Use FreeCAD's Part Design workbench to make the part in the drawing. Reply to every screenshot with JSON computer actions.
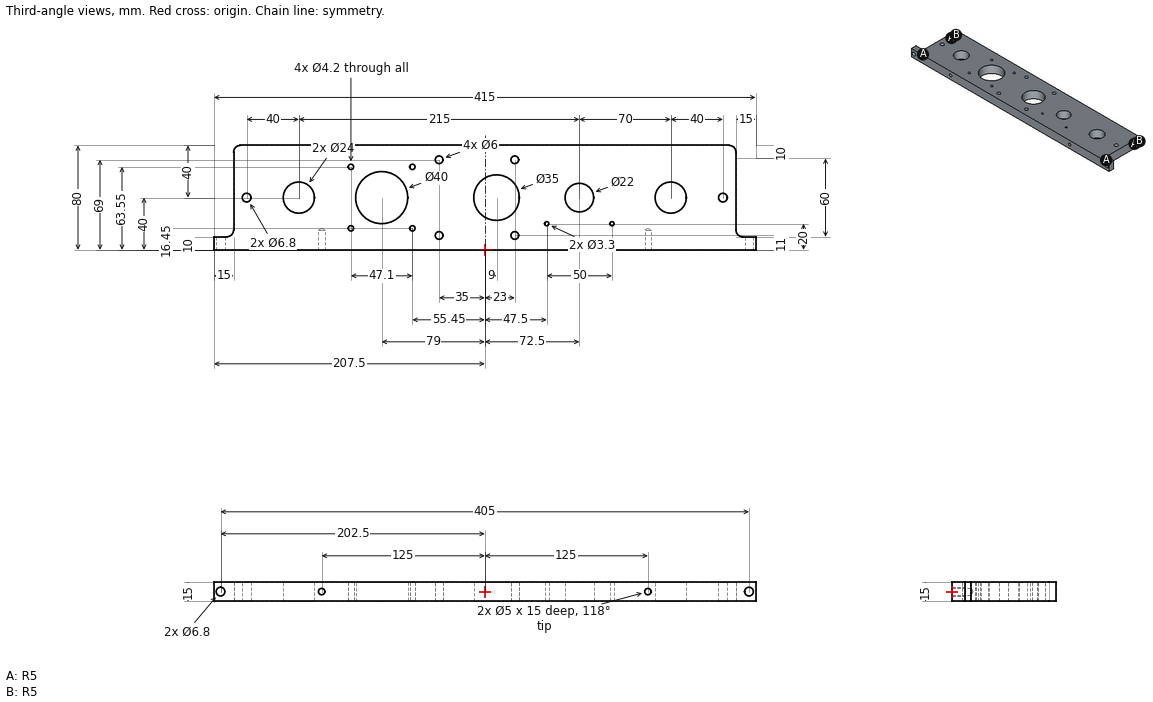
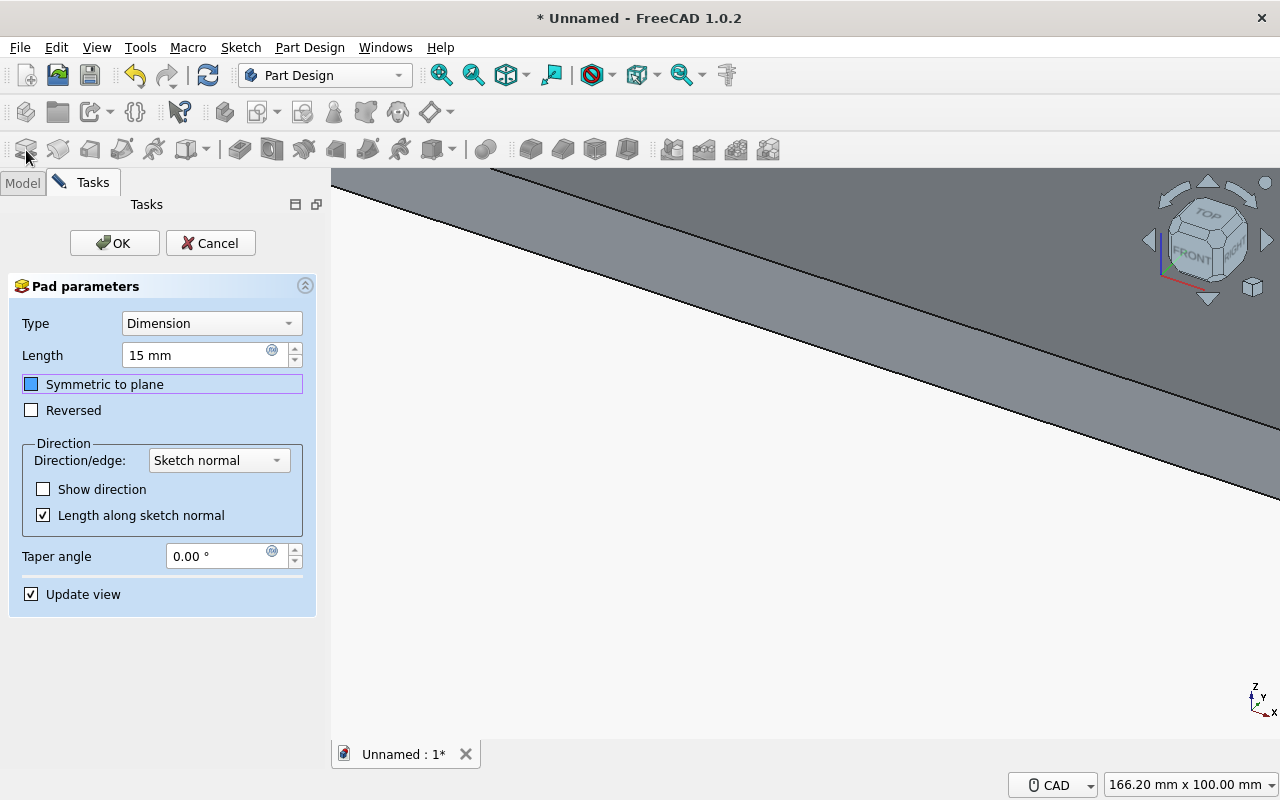
{"action": "left_click", "coordinate": [30, 384]}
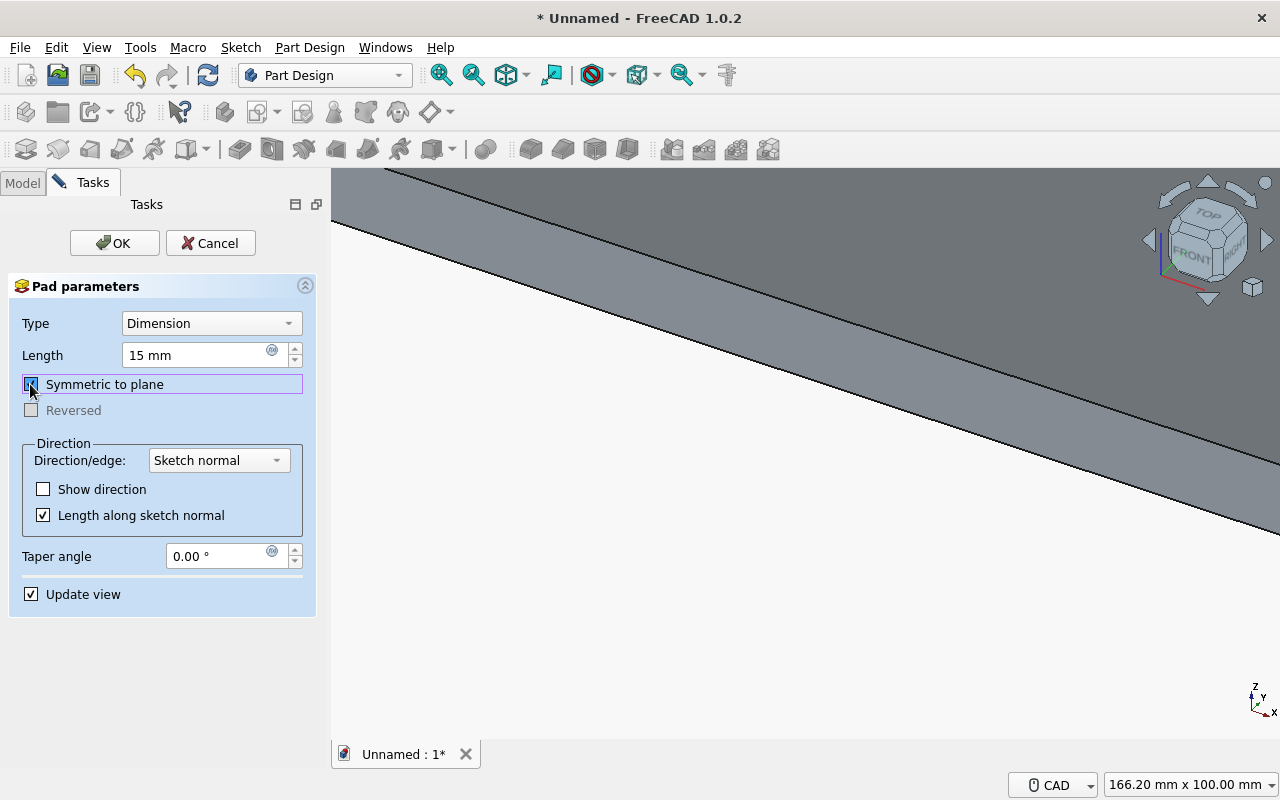
{"action": "left_click", "coordinate": [115, 243]}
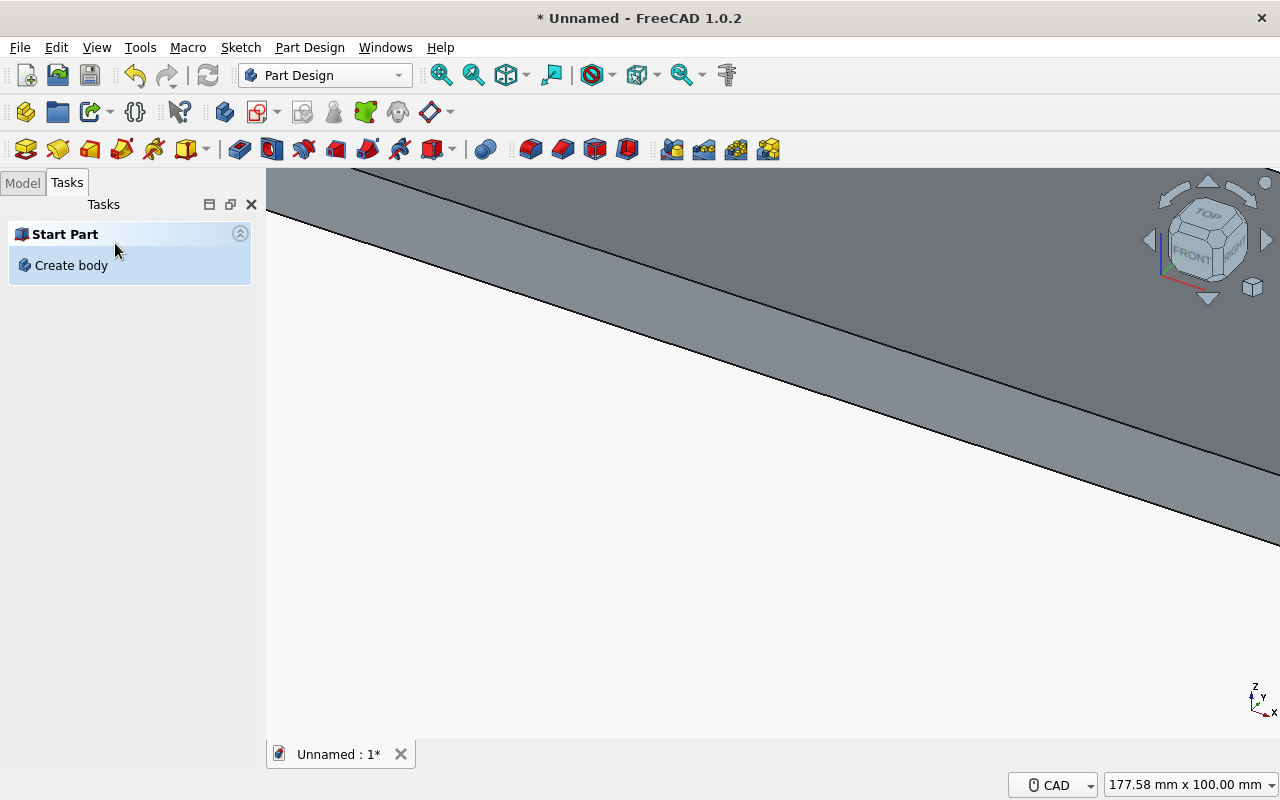
{"action": "left_click", "coordinate": [442, 76]}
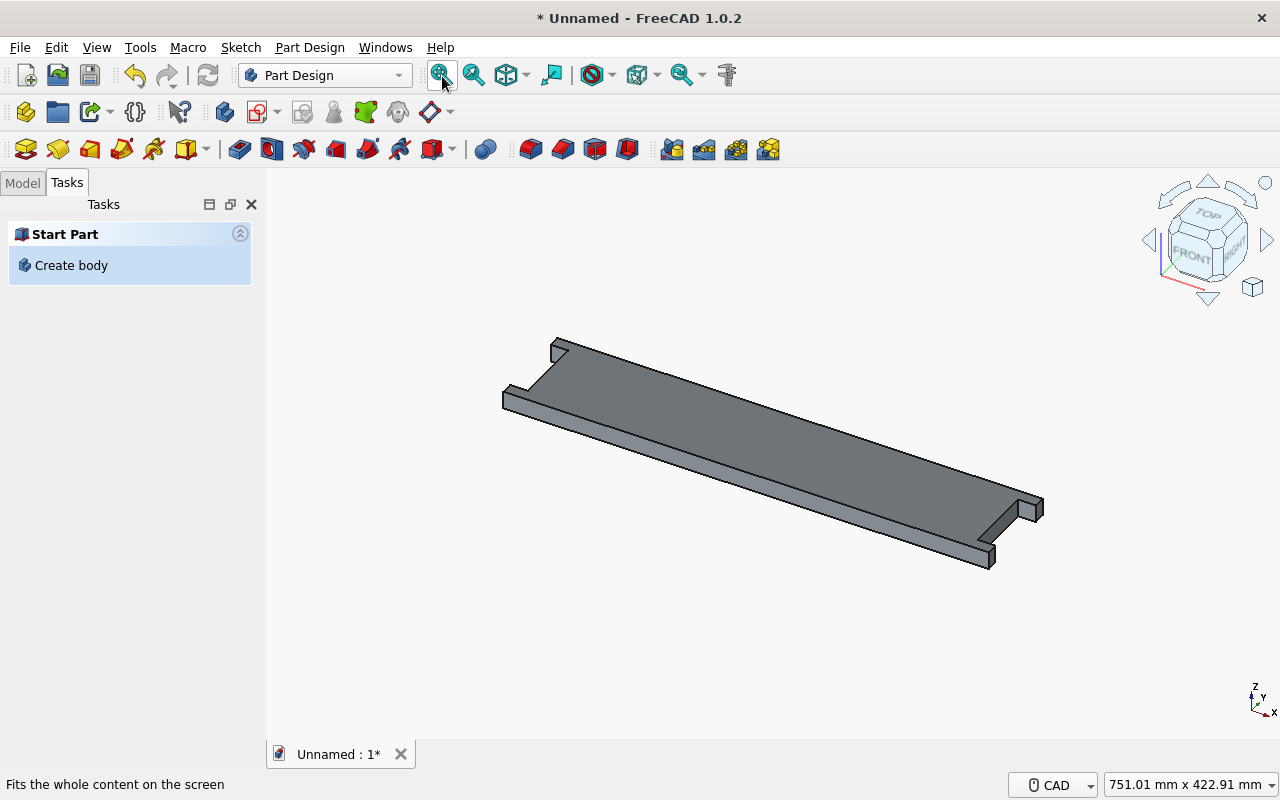
{"action": "left_click", "coordinate": [912, 490]}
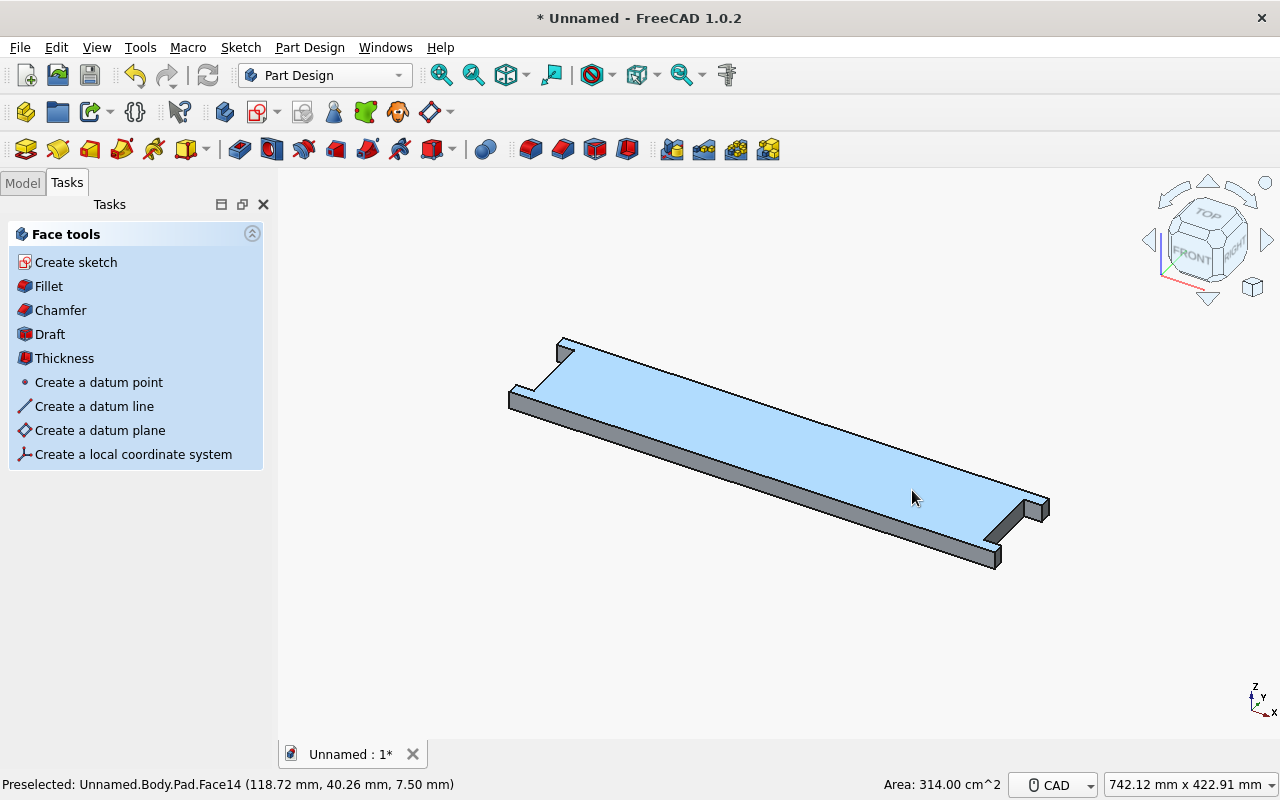
{"action": "left_click", "coordinate": [258, 112]}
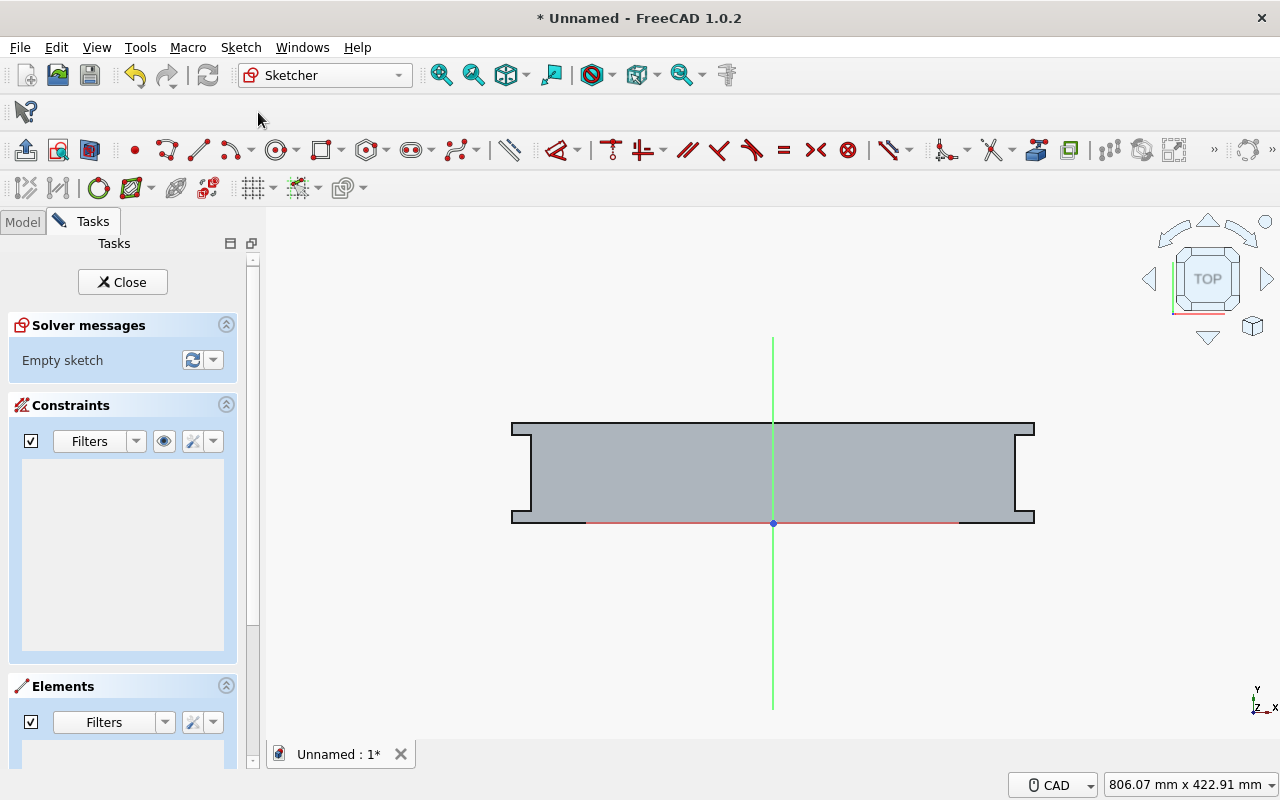
{"action": "left_click", "coordinate": [276, 150]}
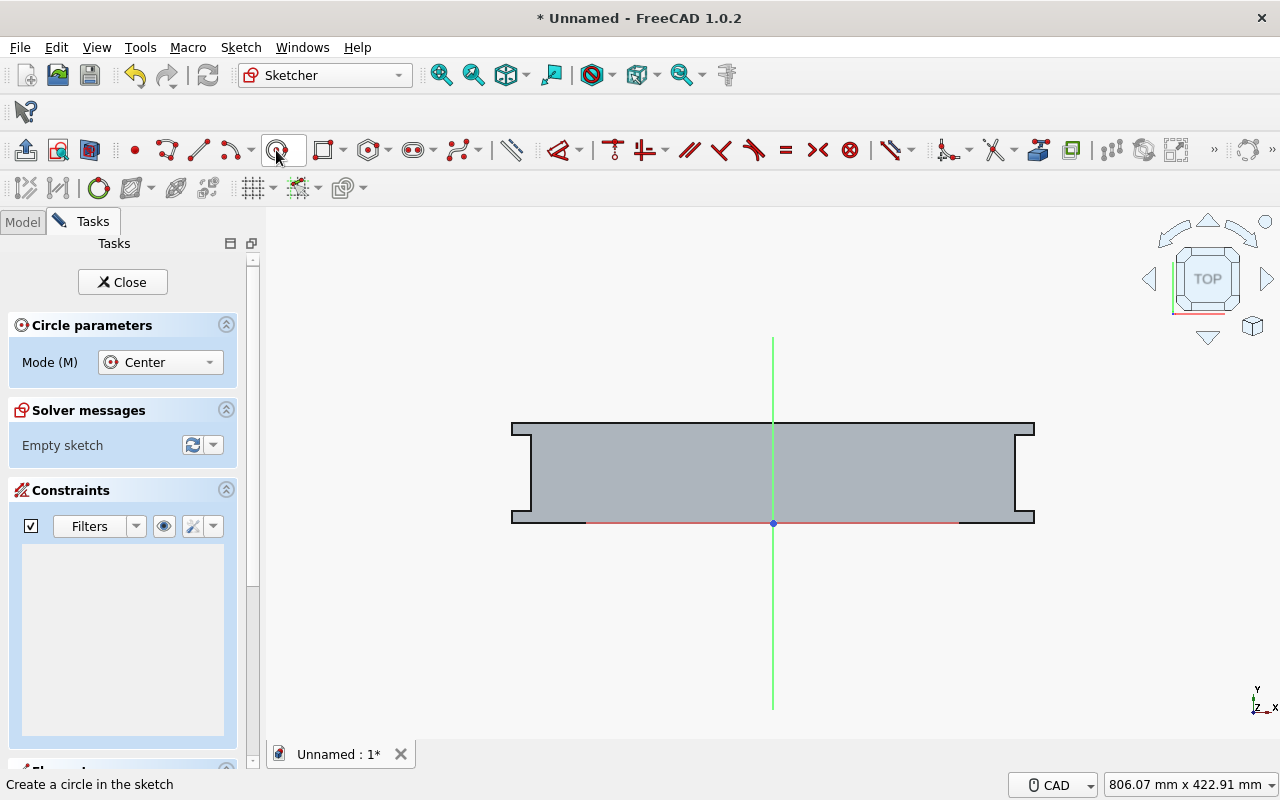
{"action": "scroll", "coordinate": [594, 473], "scroll_direction": "up", "scroll_amount": 3}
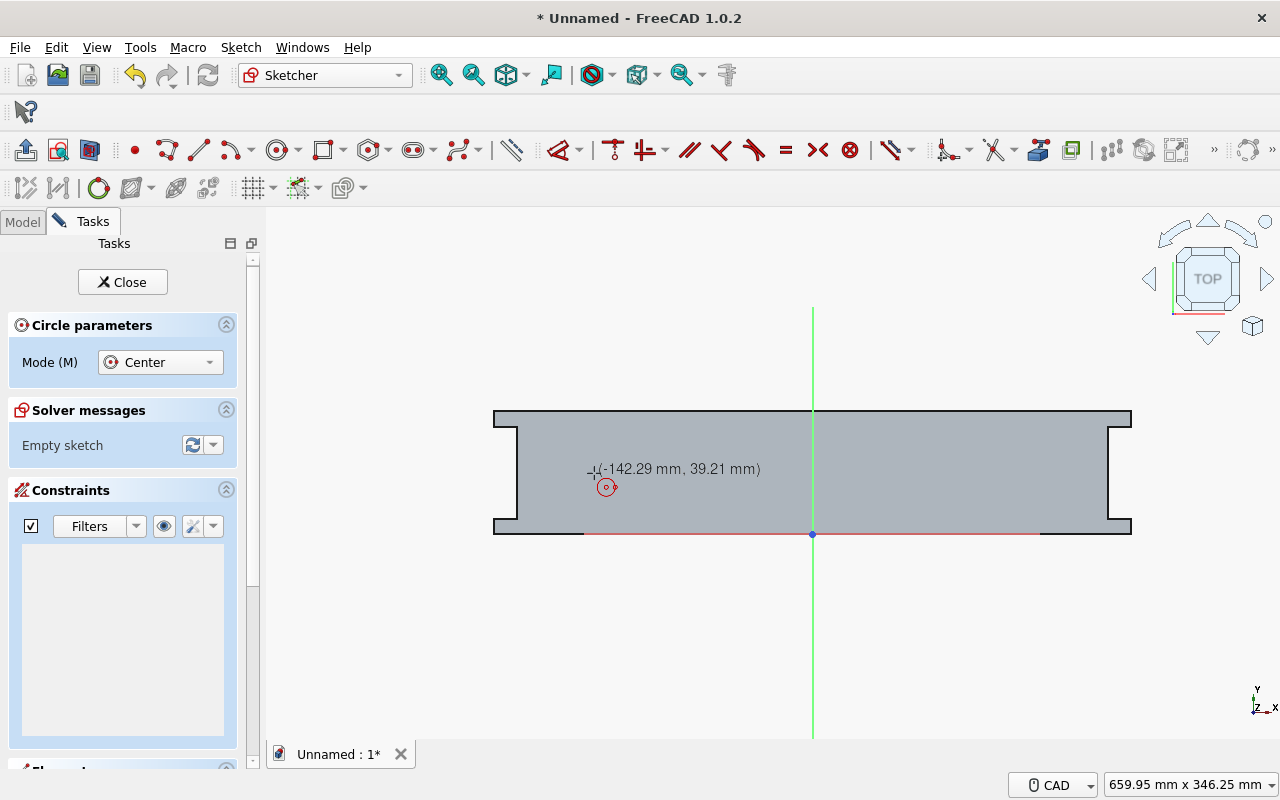
{"action": "left_click", "coordinate": [593, 473]}
{"action": "left_click", "coordinate": [613, 453]}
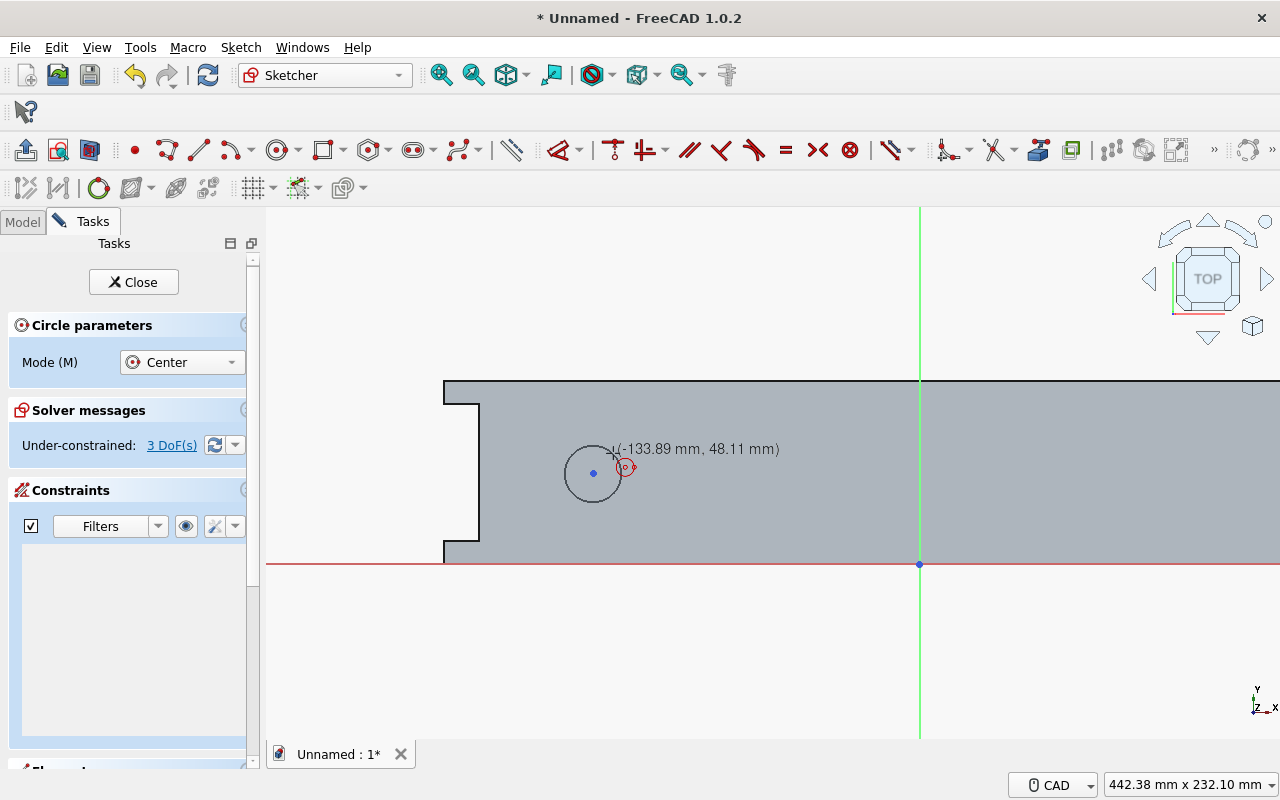
{"action": "left_click", "coordinate": [941, 473]}
{"action": "left_click", "coordinate": [969, 444]}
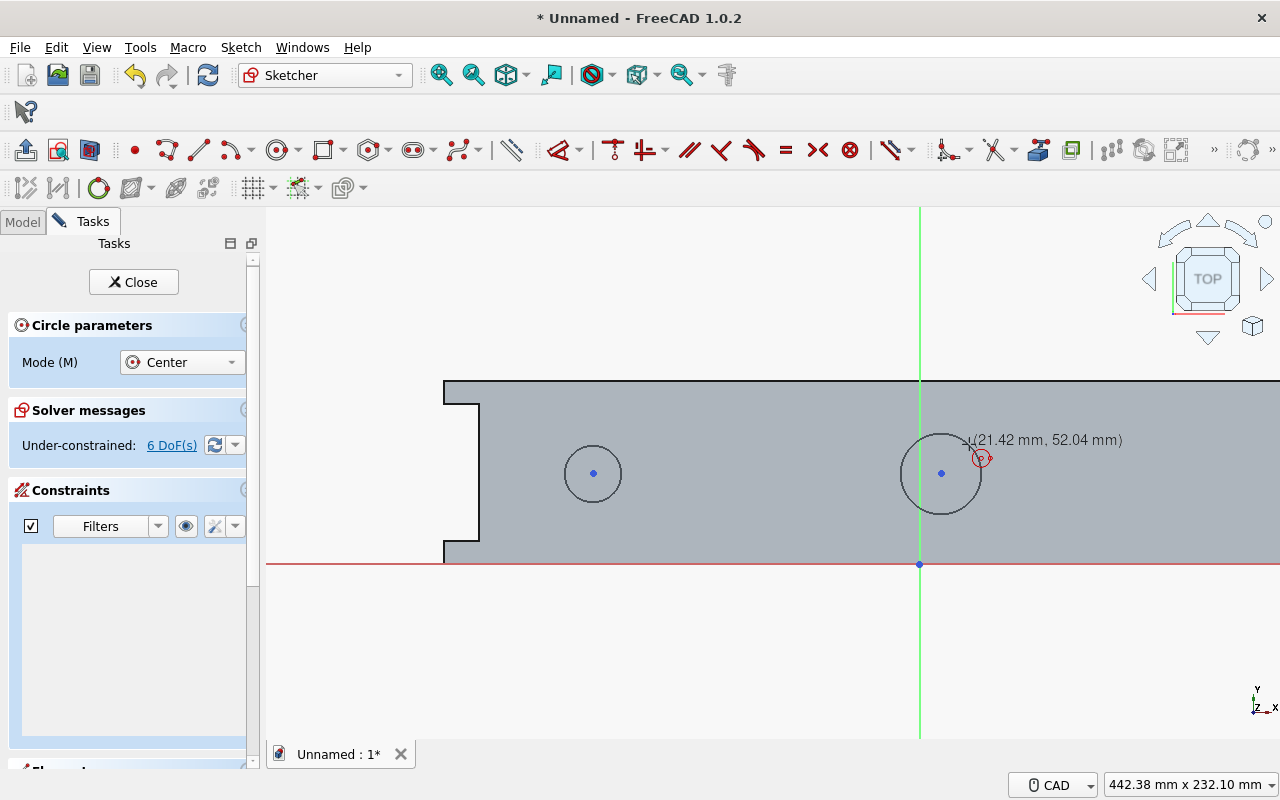
{"action": "left_click", "coordinate": [1086, 473]}
{"action": "left_click", "coordinate": [1104, 455]}